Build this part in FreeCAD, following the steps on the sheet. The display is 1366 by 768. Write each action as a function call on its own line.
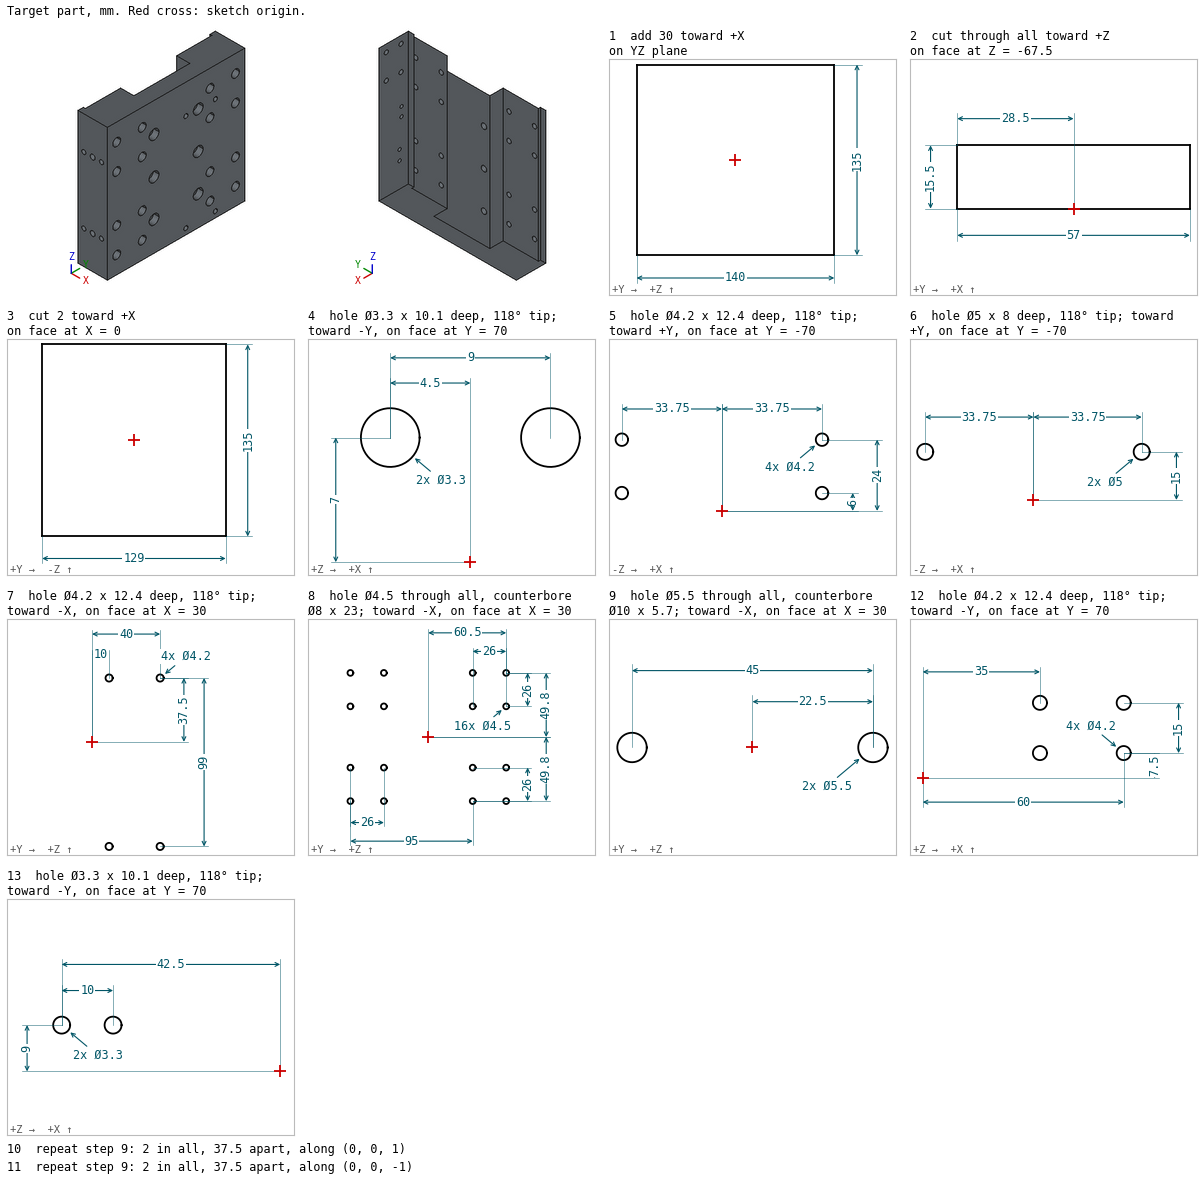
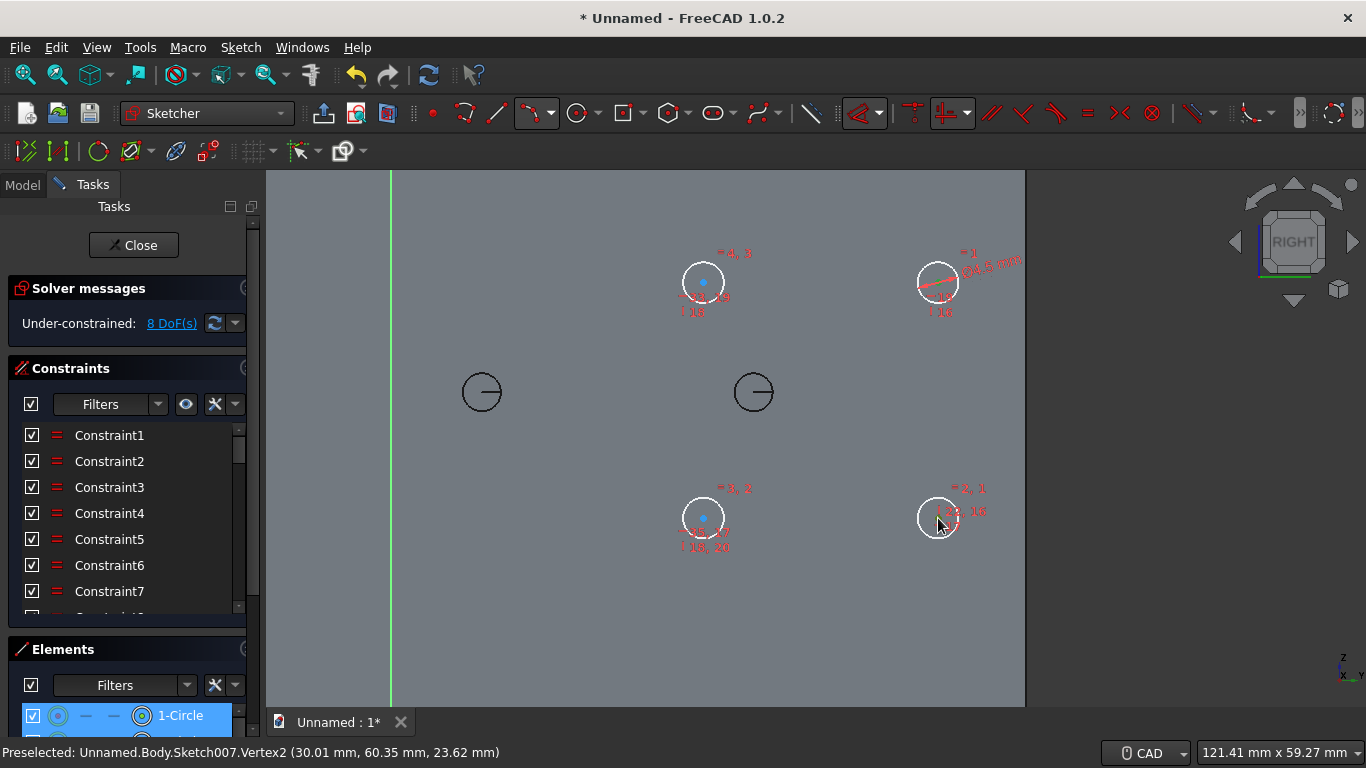
key(i)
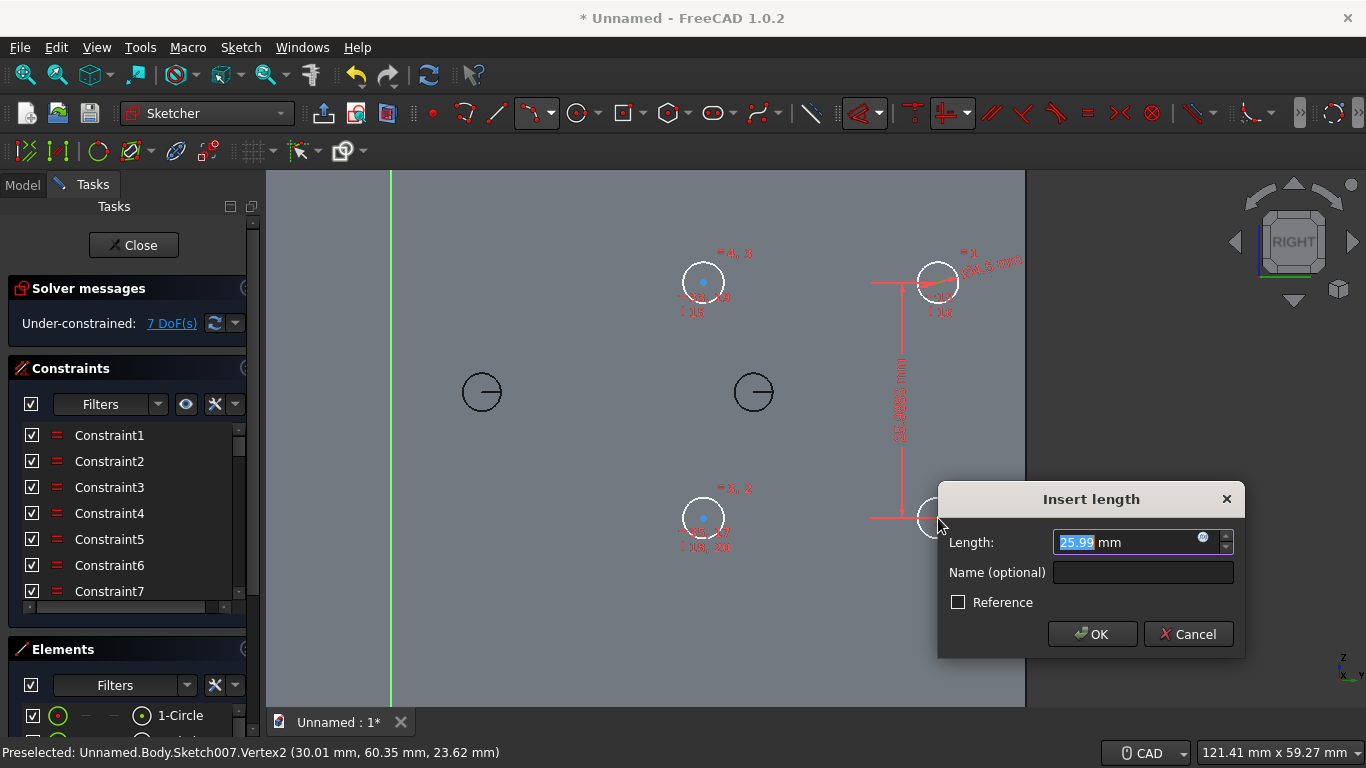
text(26)
key(Return)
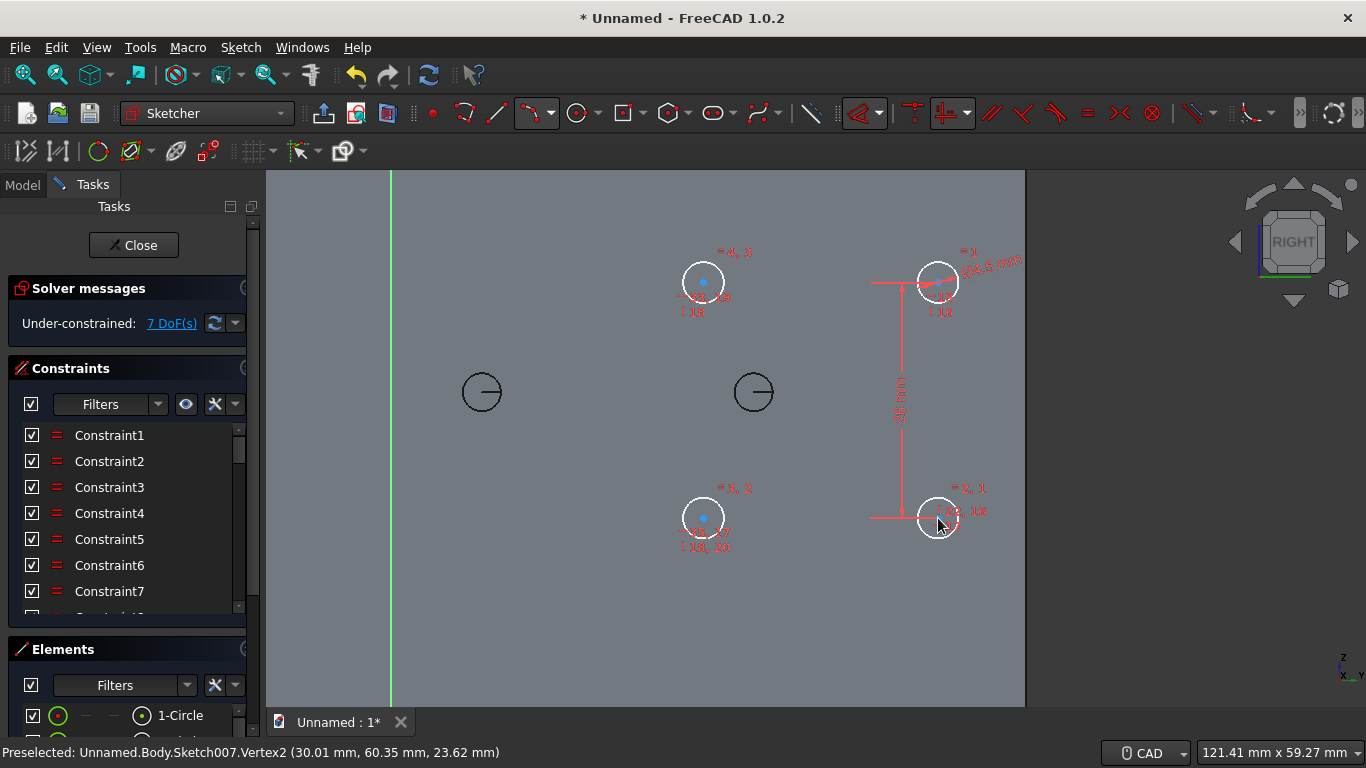
click(938, 518)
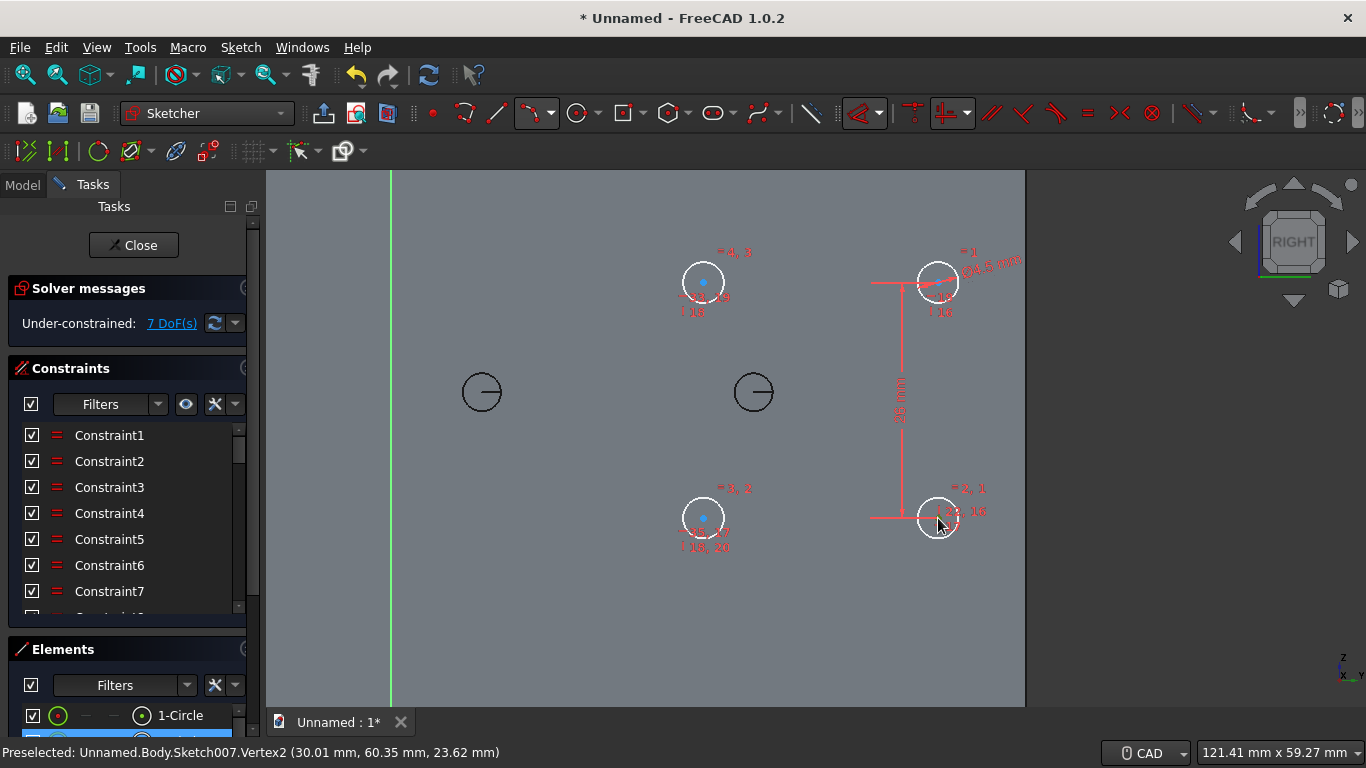
click(704, 518)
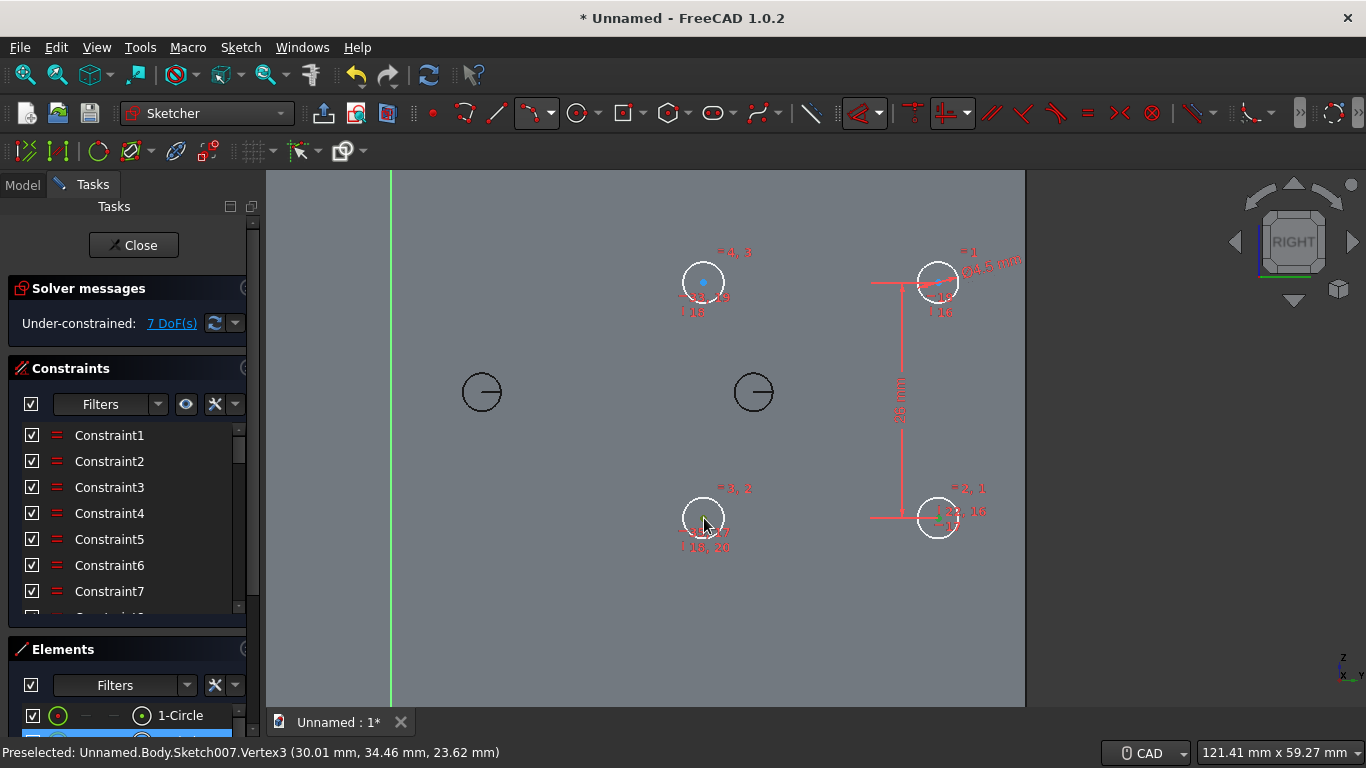
key(l)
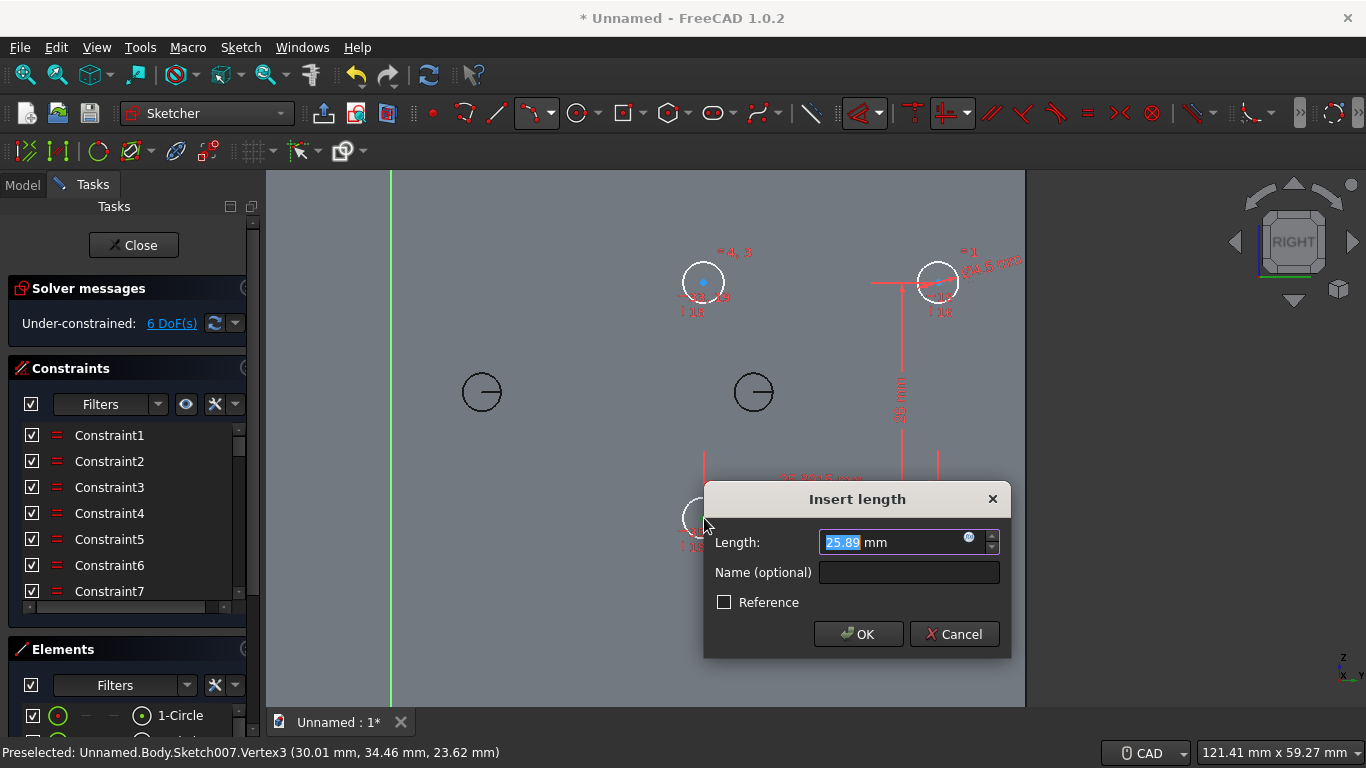
text(26)
key(Return)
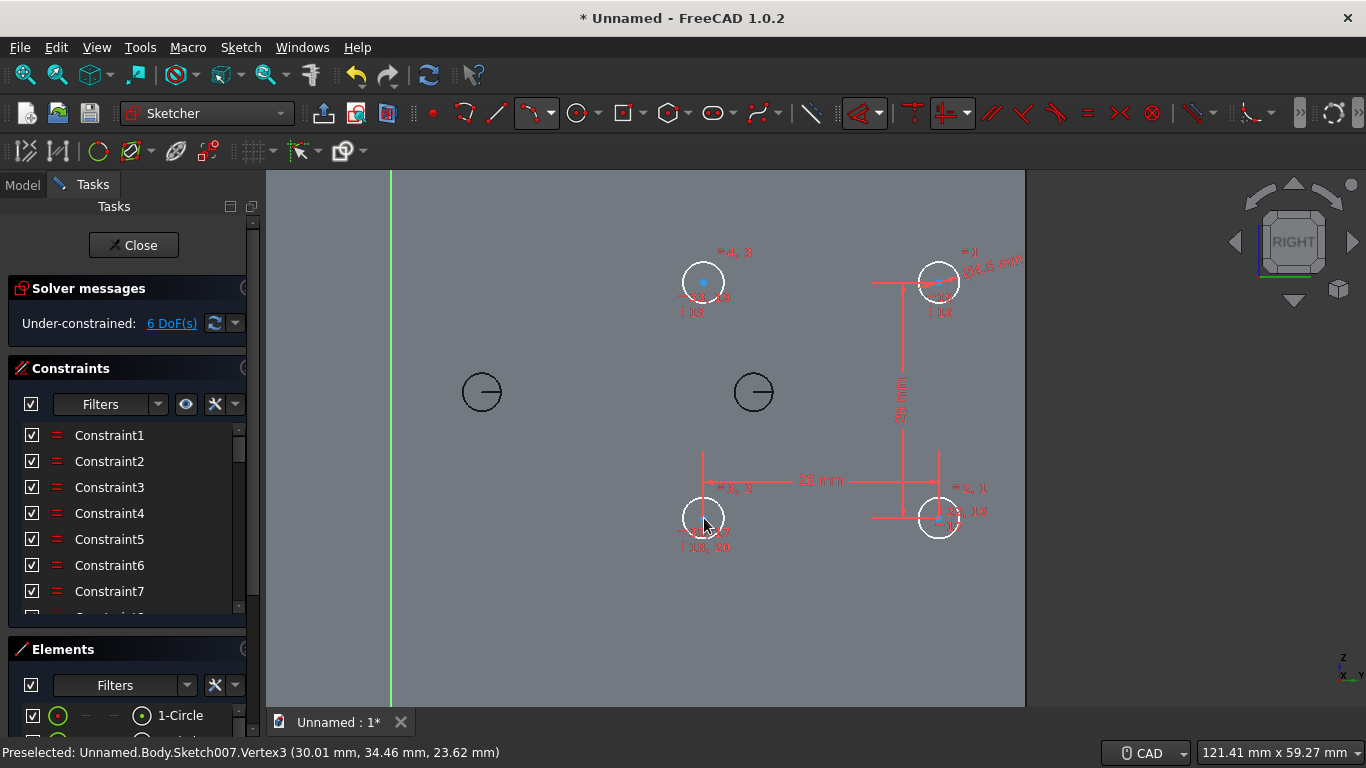
scroll(955, 268, down, 5)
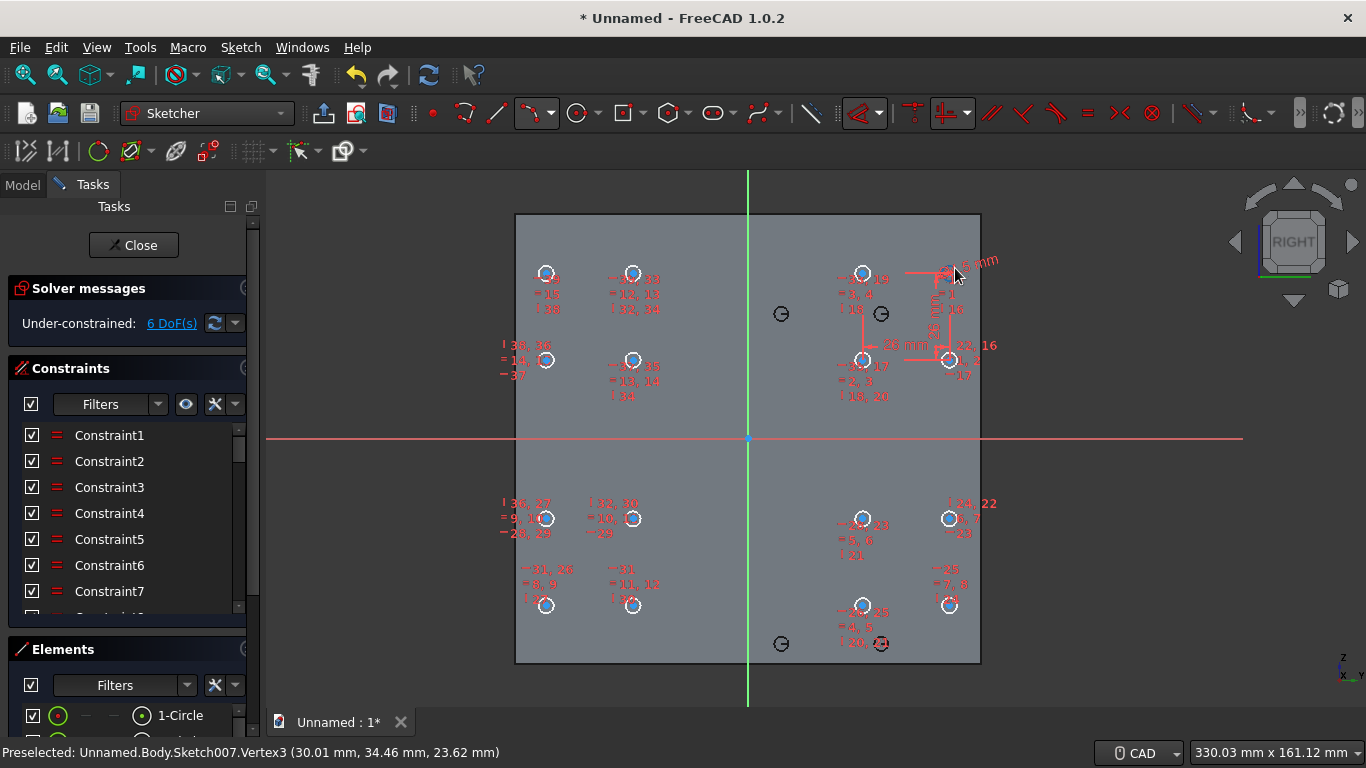
click(863, 606)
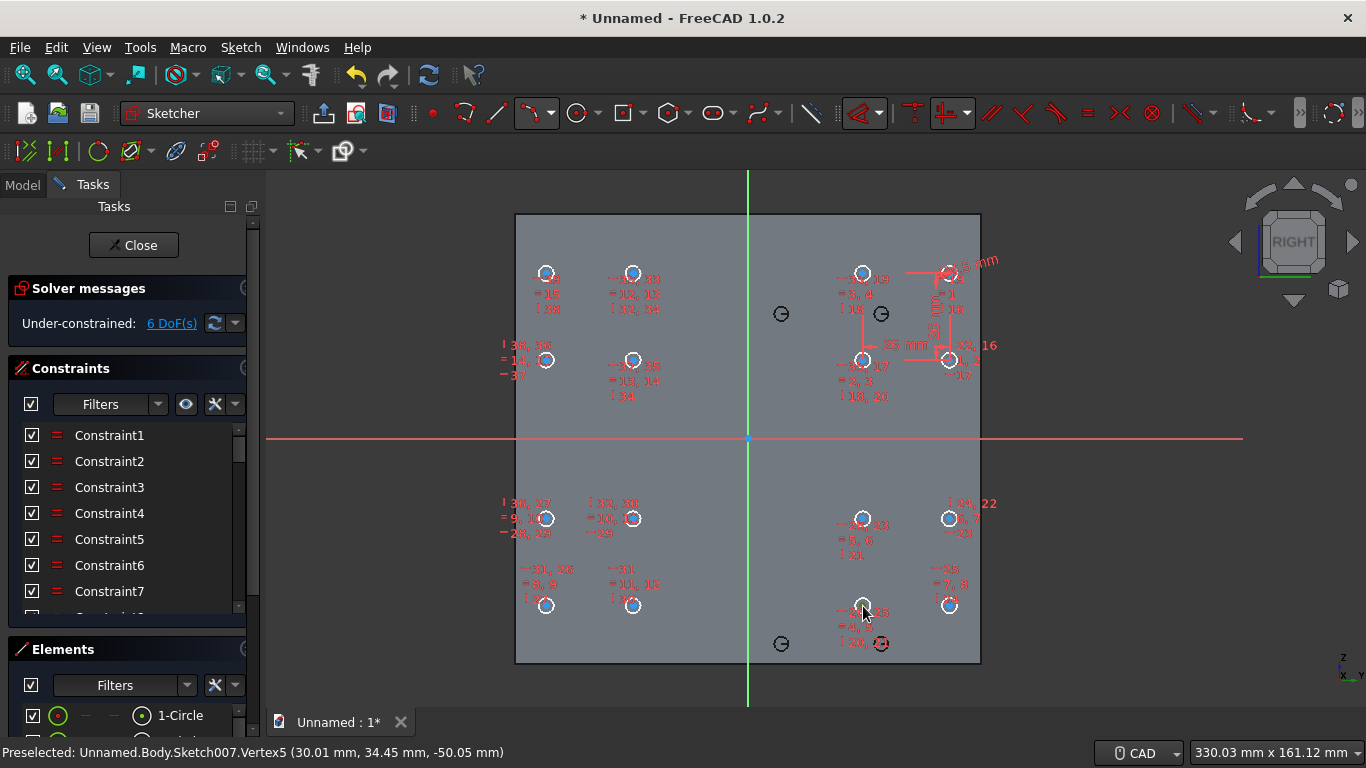
click(863, 519)